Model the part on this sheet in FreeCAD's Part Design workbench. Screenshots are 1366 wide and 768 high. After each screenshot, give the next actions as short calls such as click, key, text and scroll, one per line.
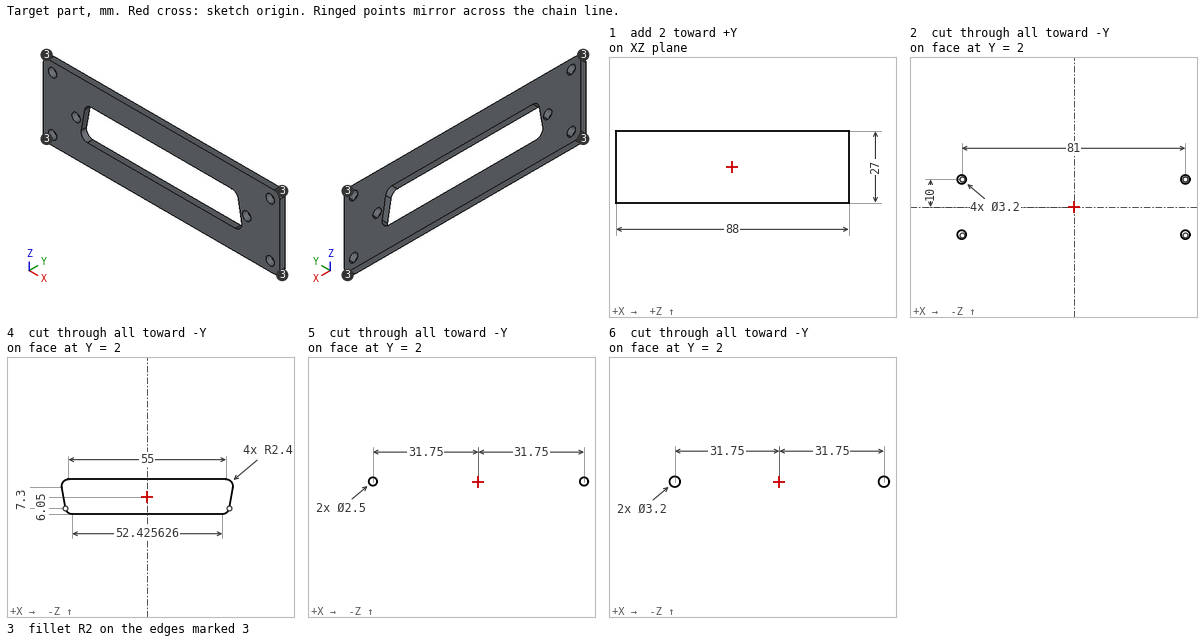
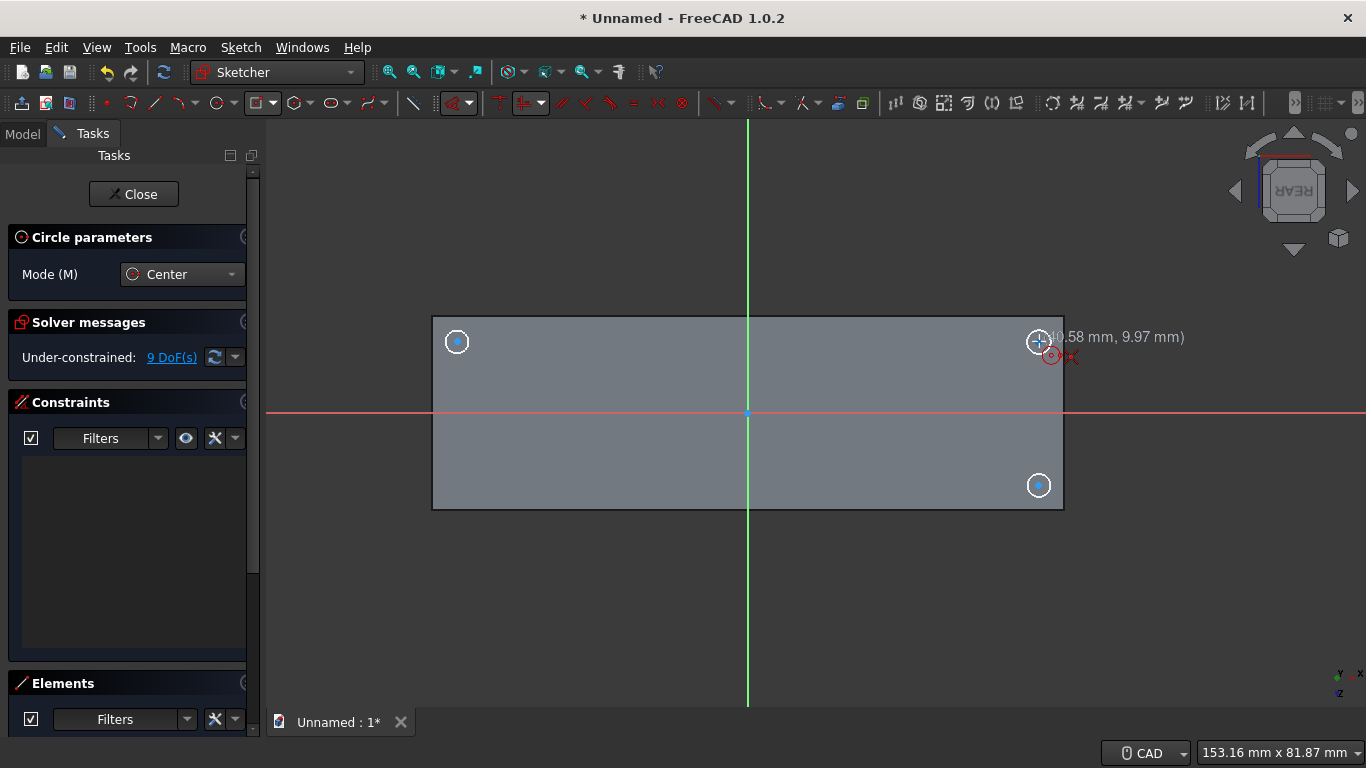
scroll(457, 485, up, 4)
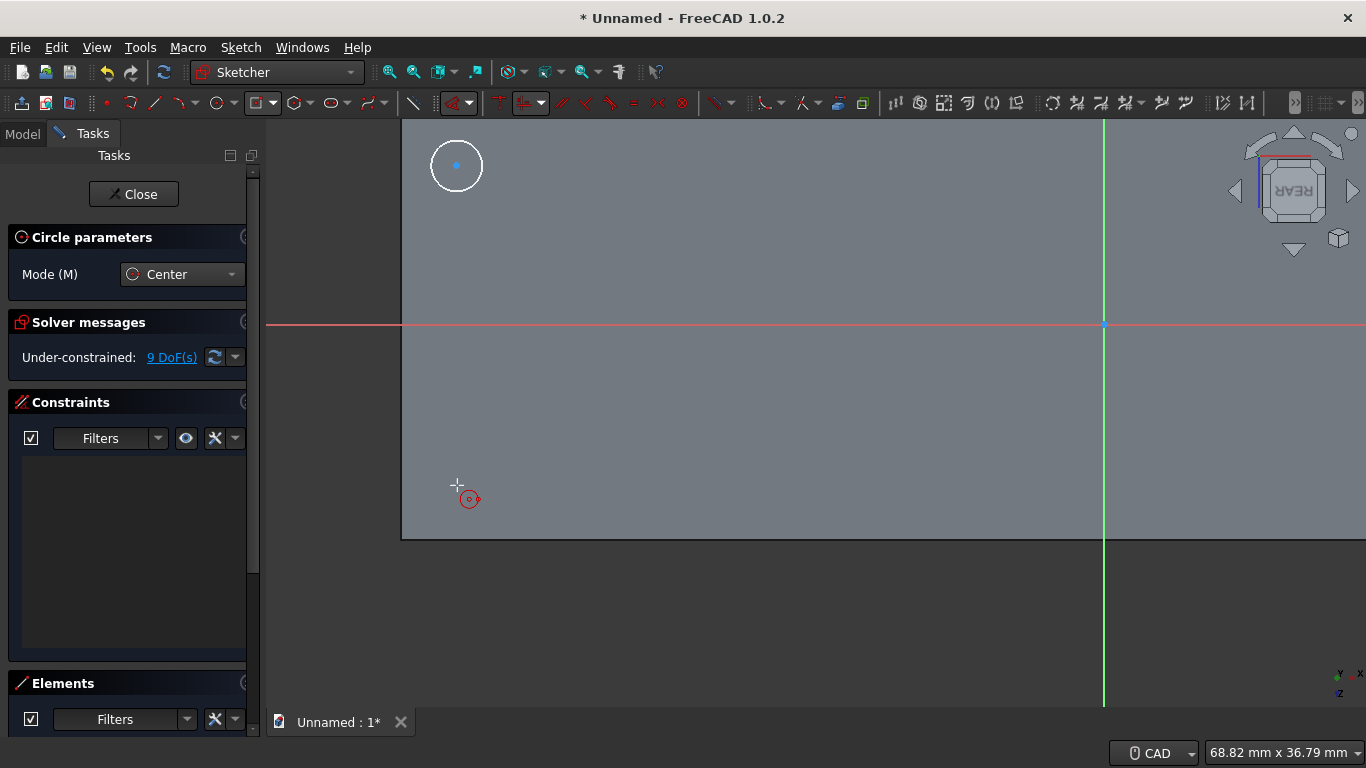
click(457, 484)
click(475, 466)
key(Escape)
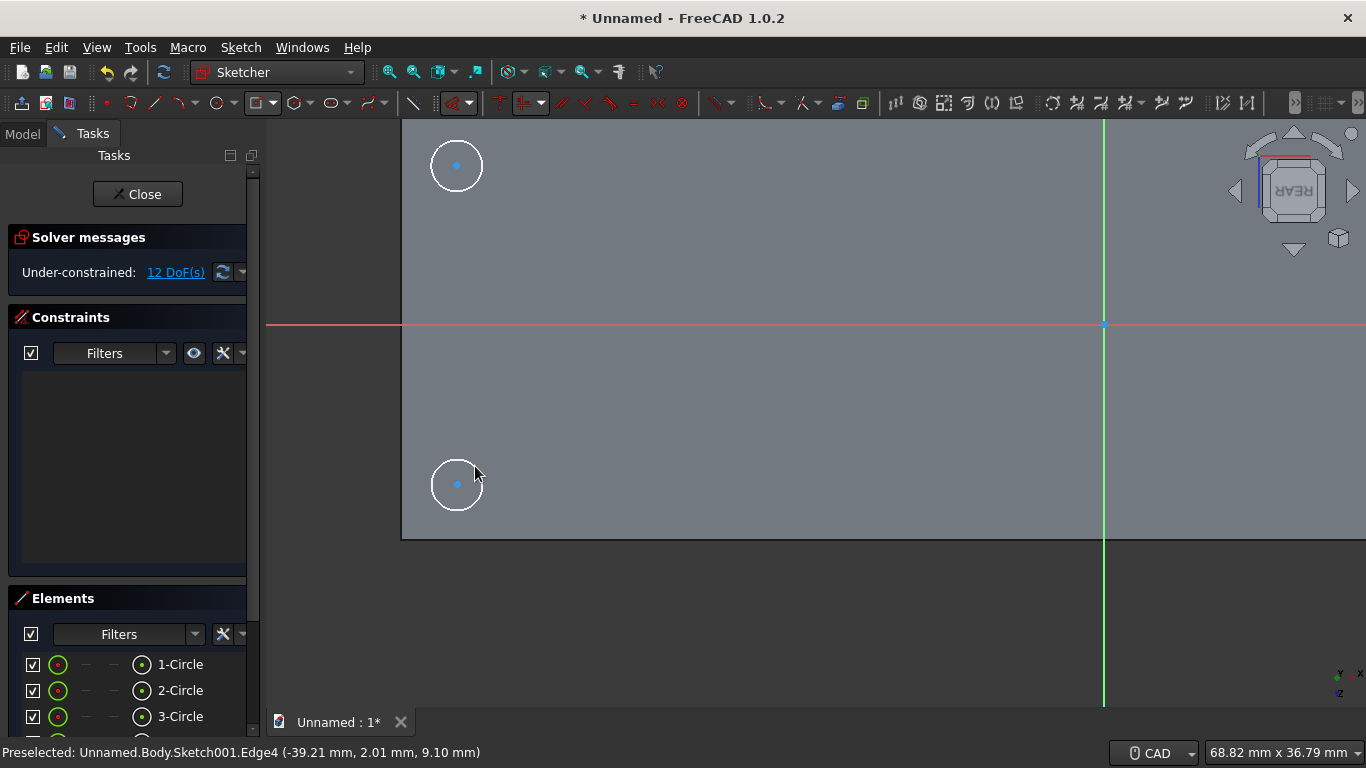
click(475, 148)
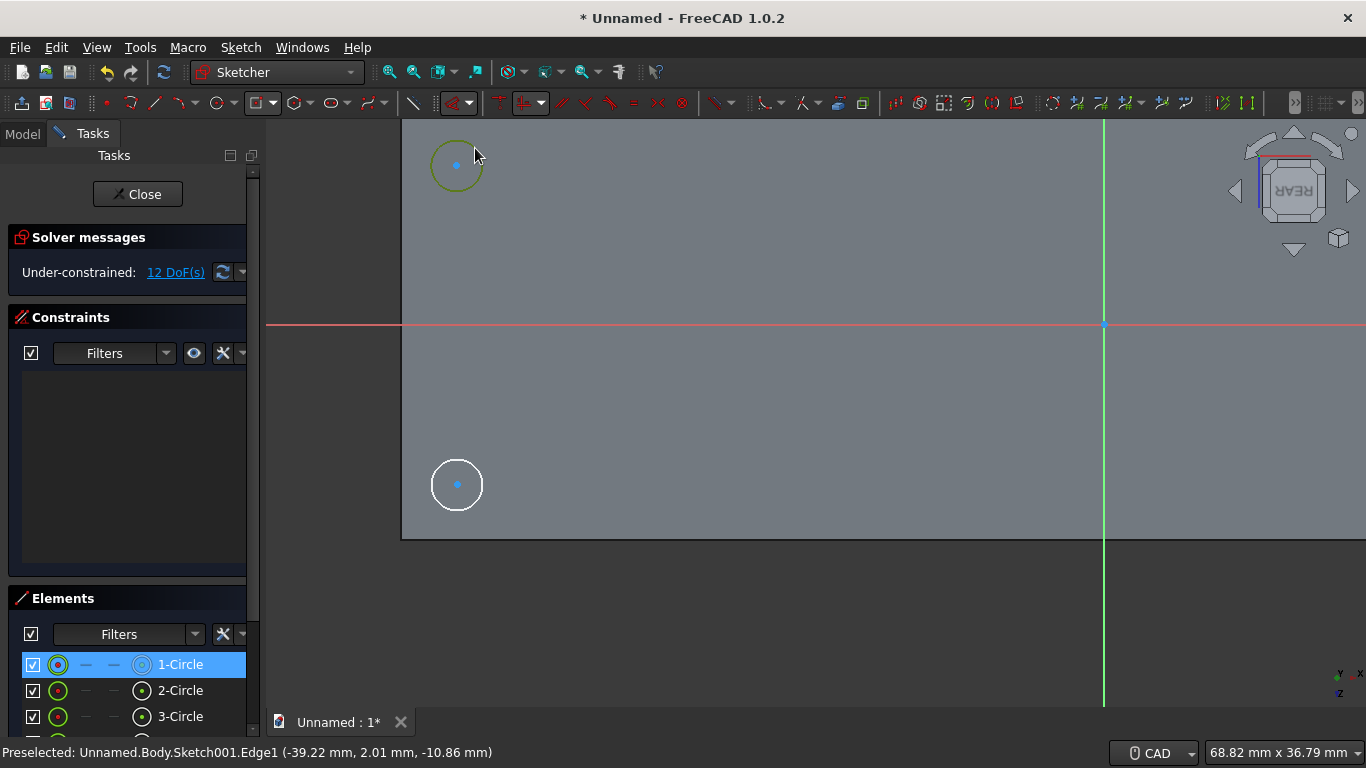
scroll(456, 485, down, 4)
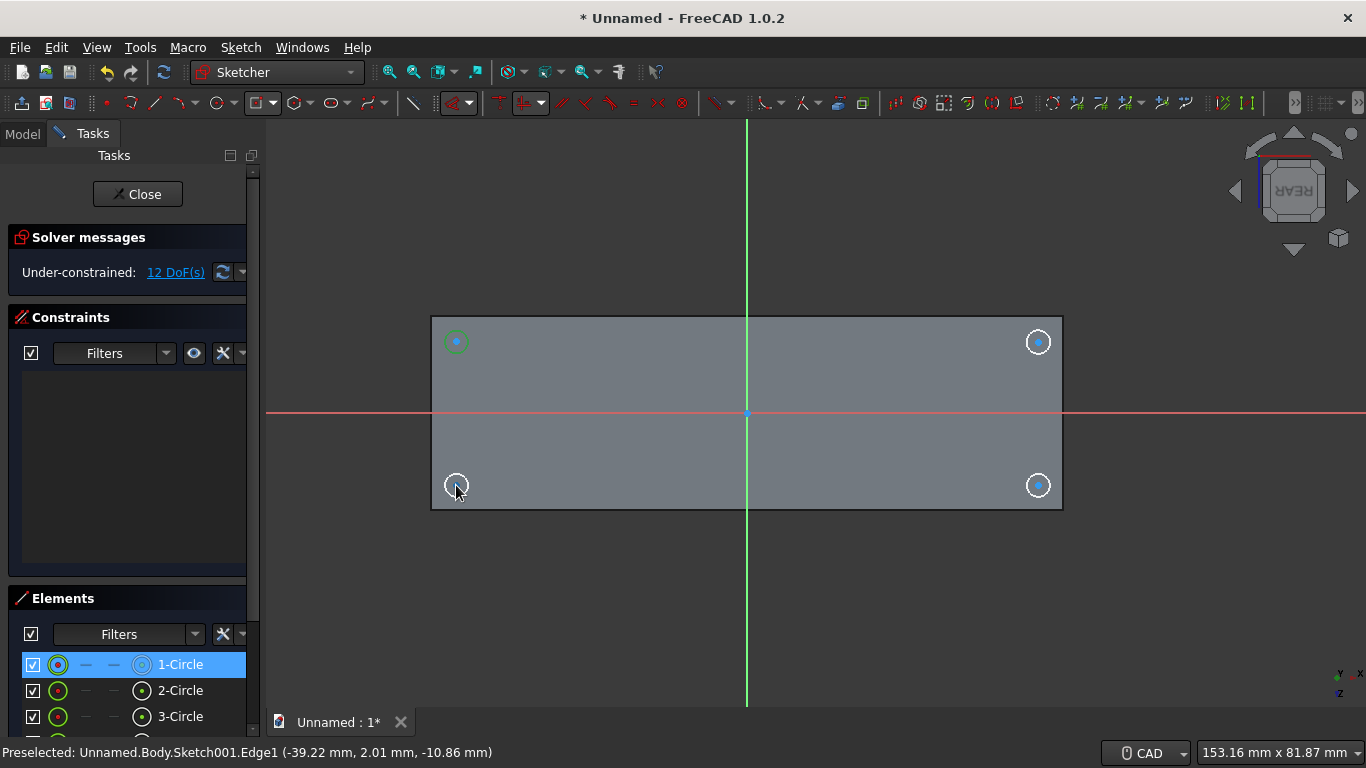
click(1047, 334)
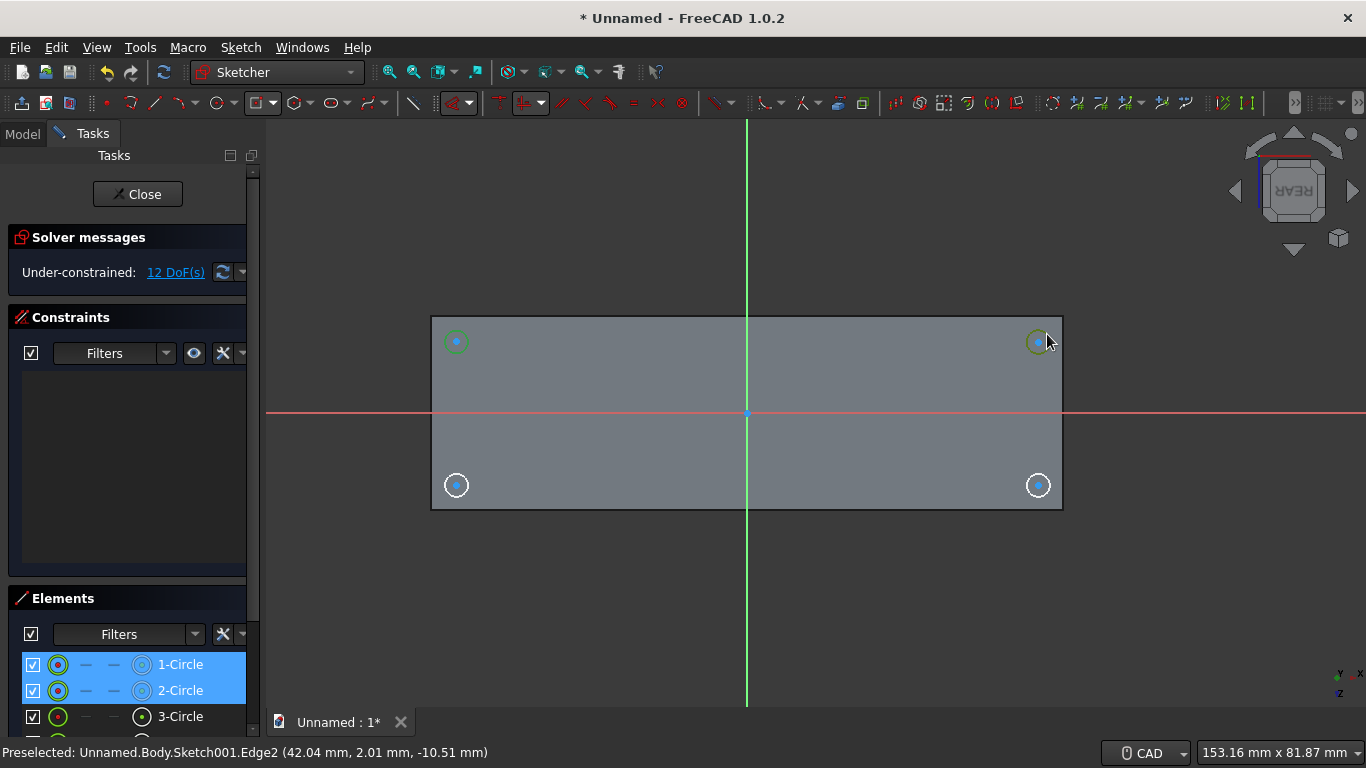
click(1046, 477)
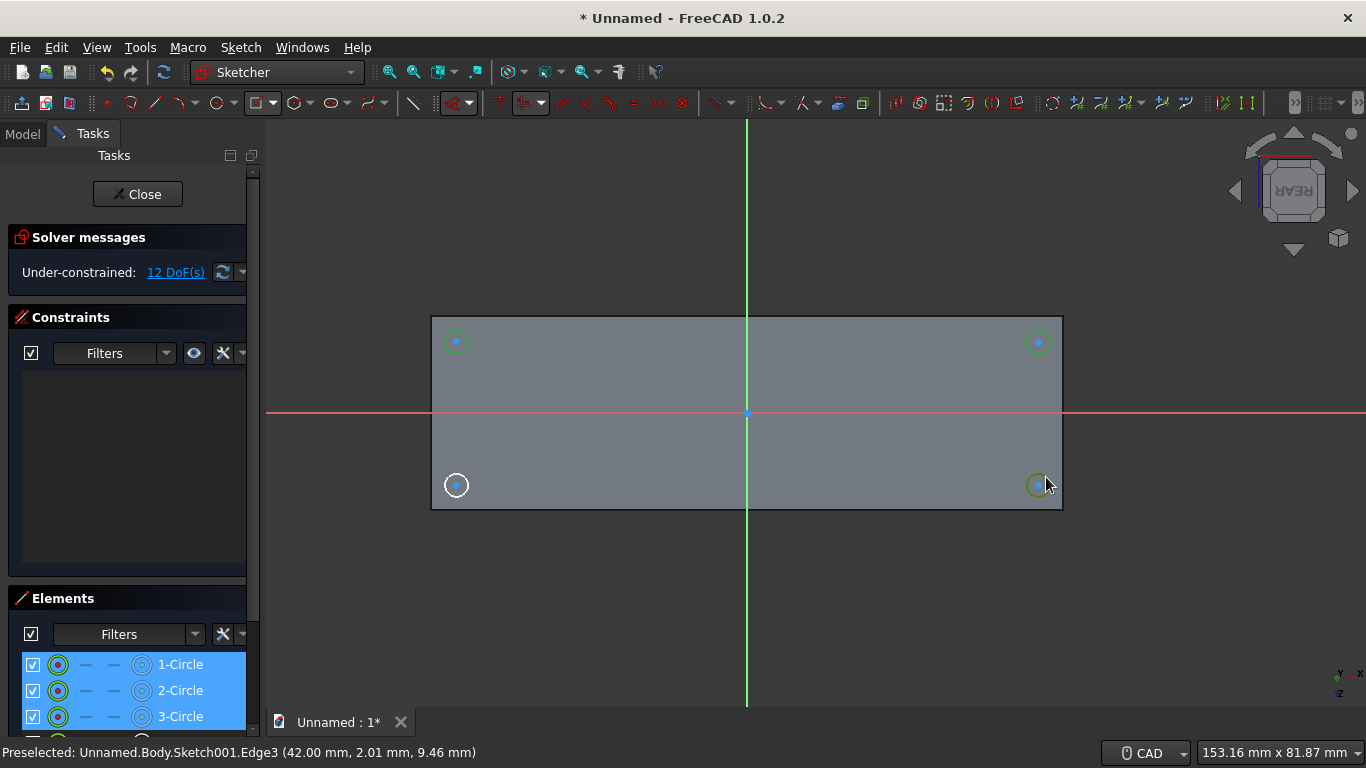
click(465, 477)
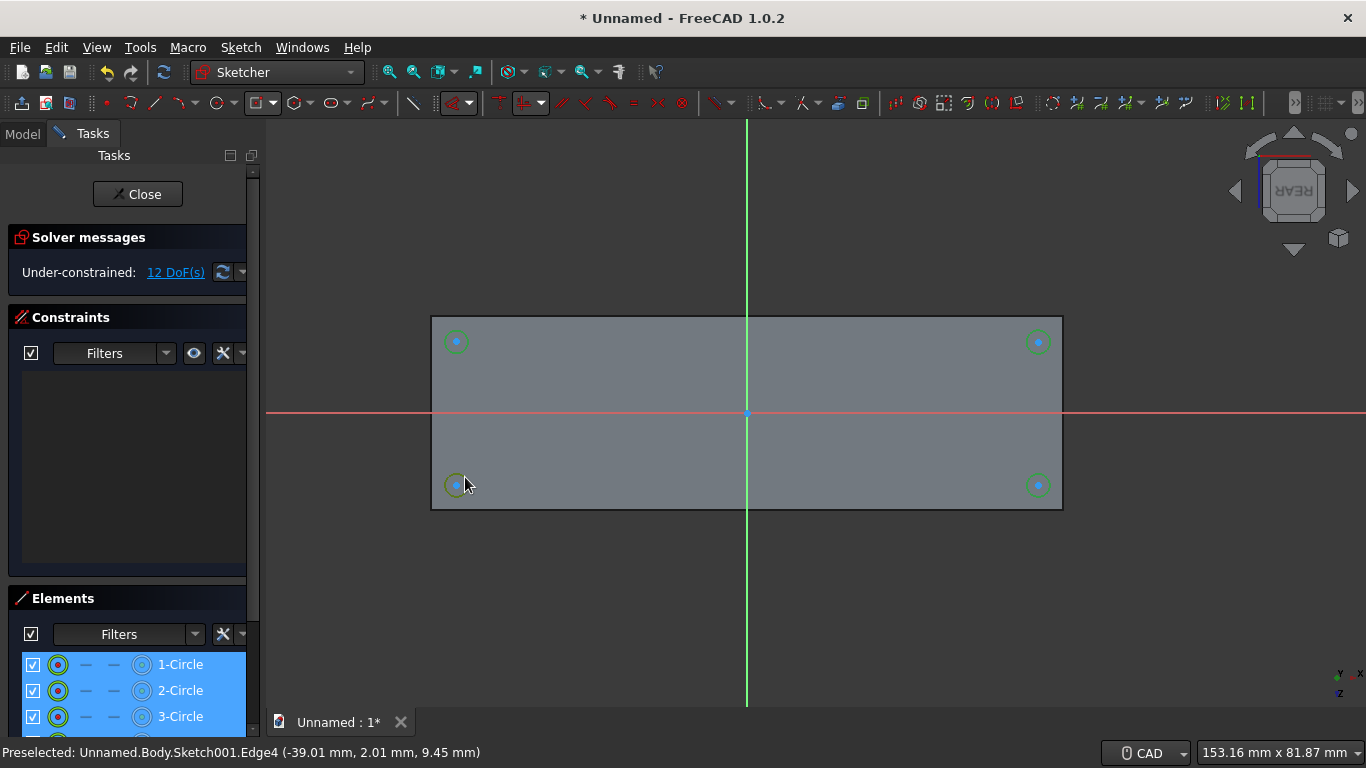
click(634, 104)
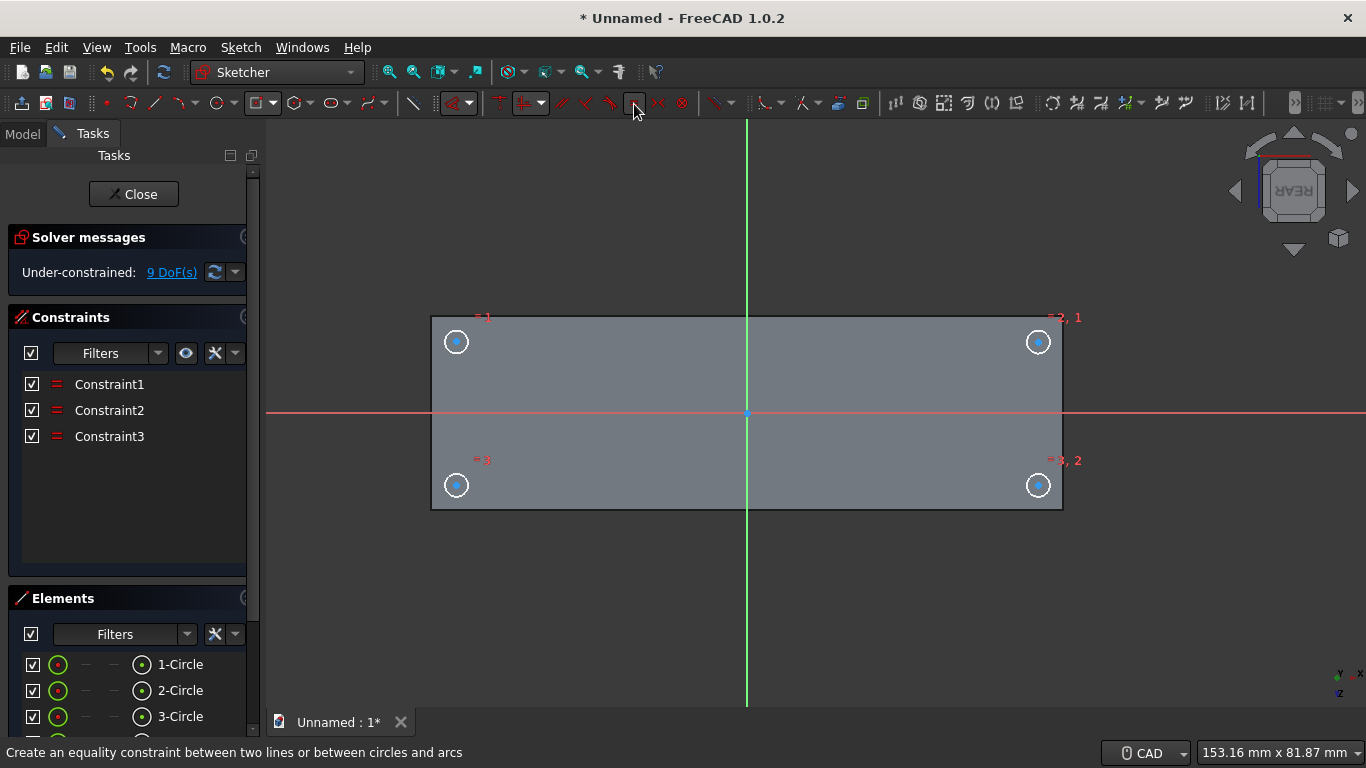
click(456, 342)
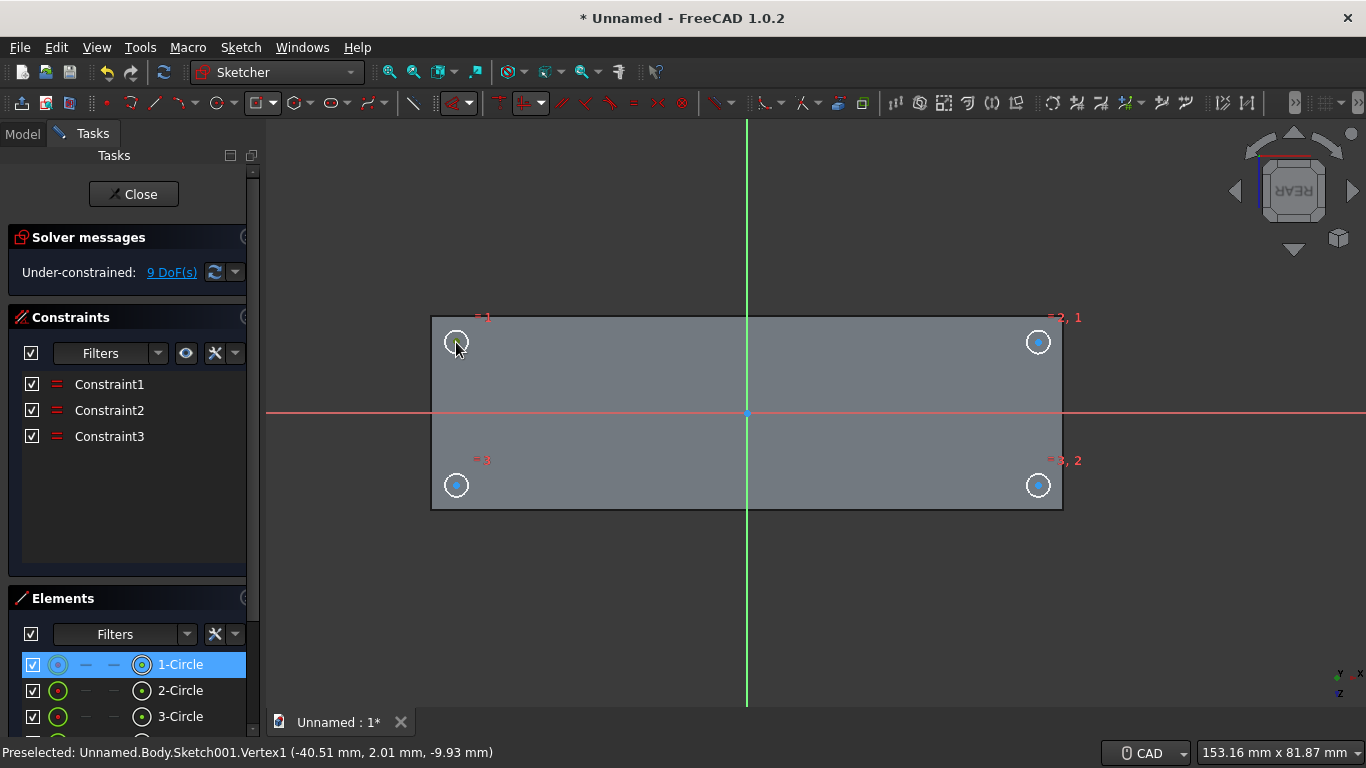
click(1038, 342)